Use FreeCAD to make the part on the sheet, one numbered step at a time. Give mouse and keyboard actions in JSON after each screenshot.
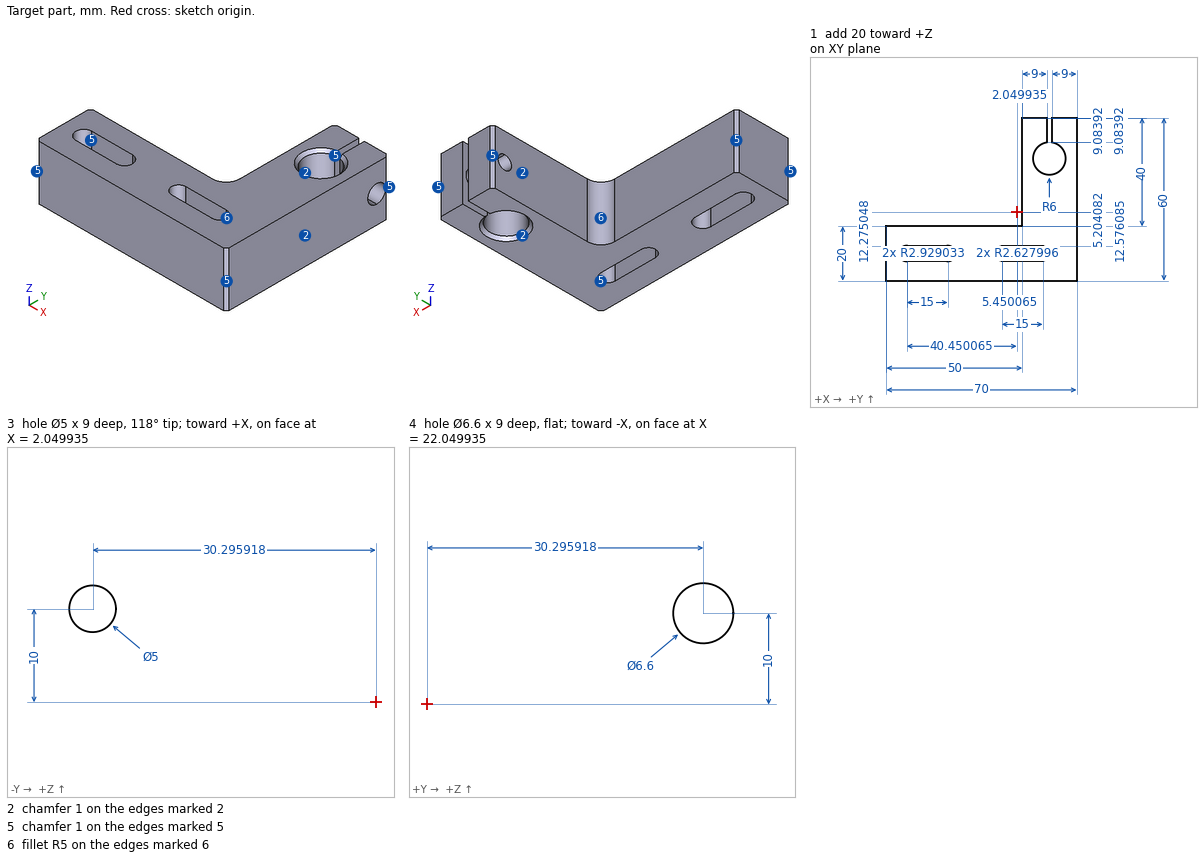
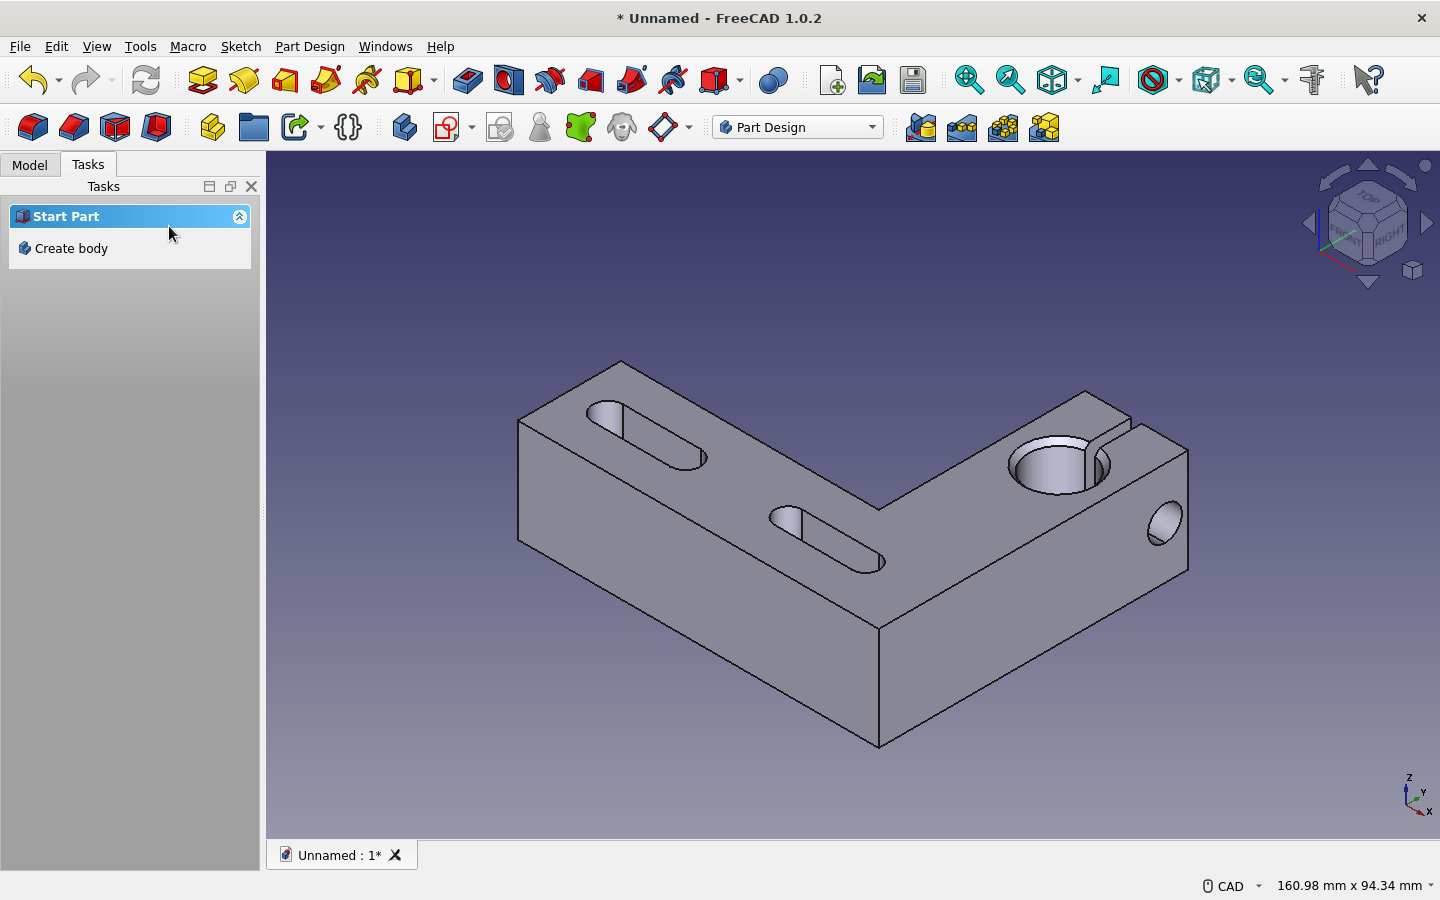
{"action": "left_click", "coordinate": [879, 688]}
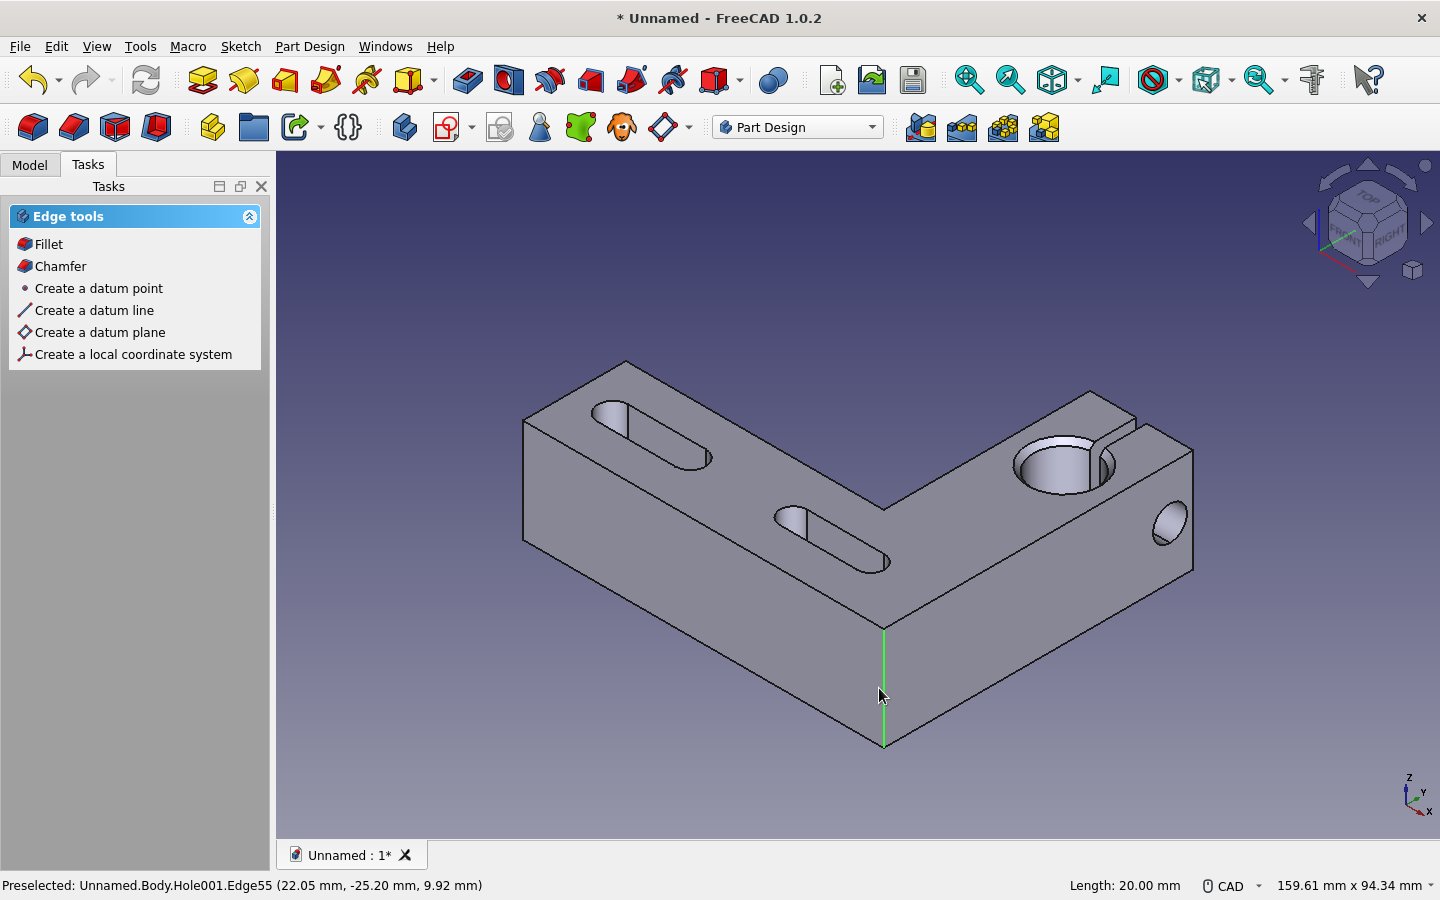
{"action": "key", "text": "2"}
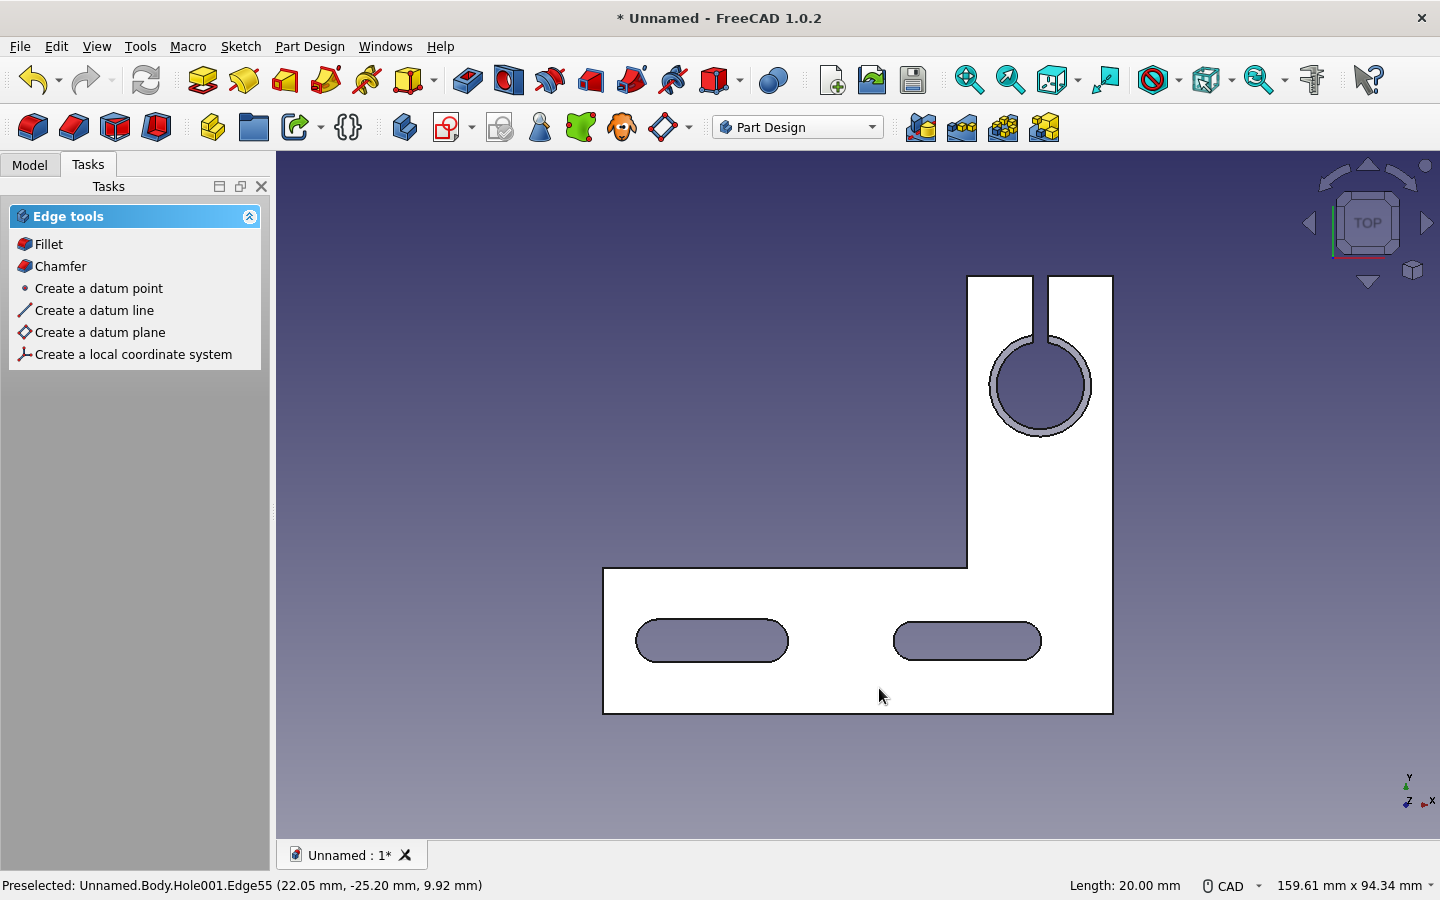
{"action": "key", "text": "0"}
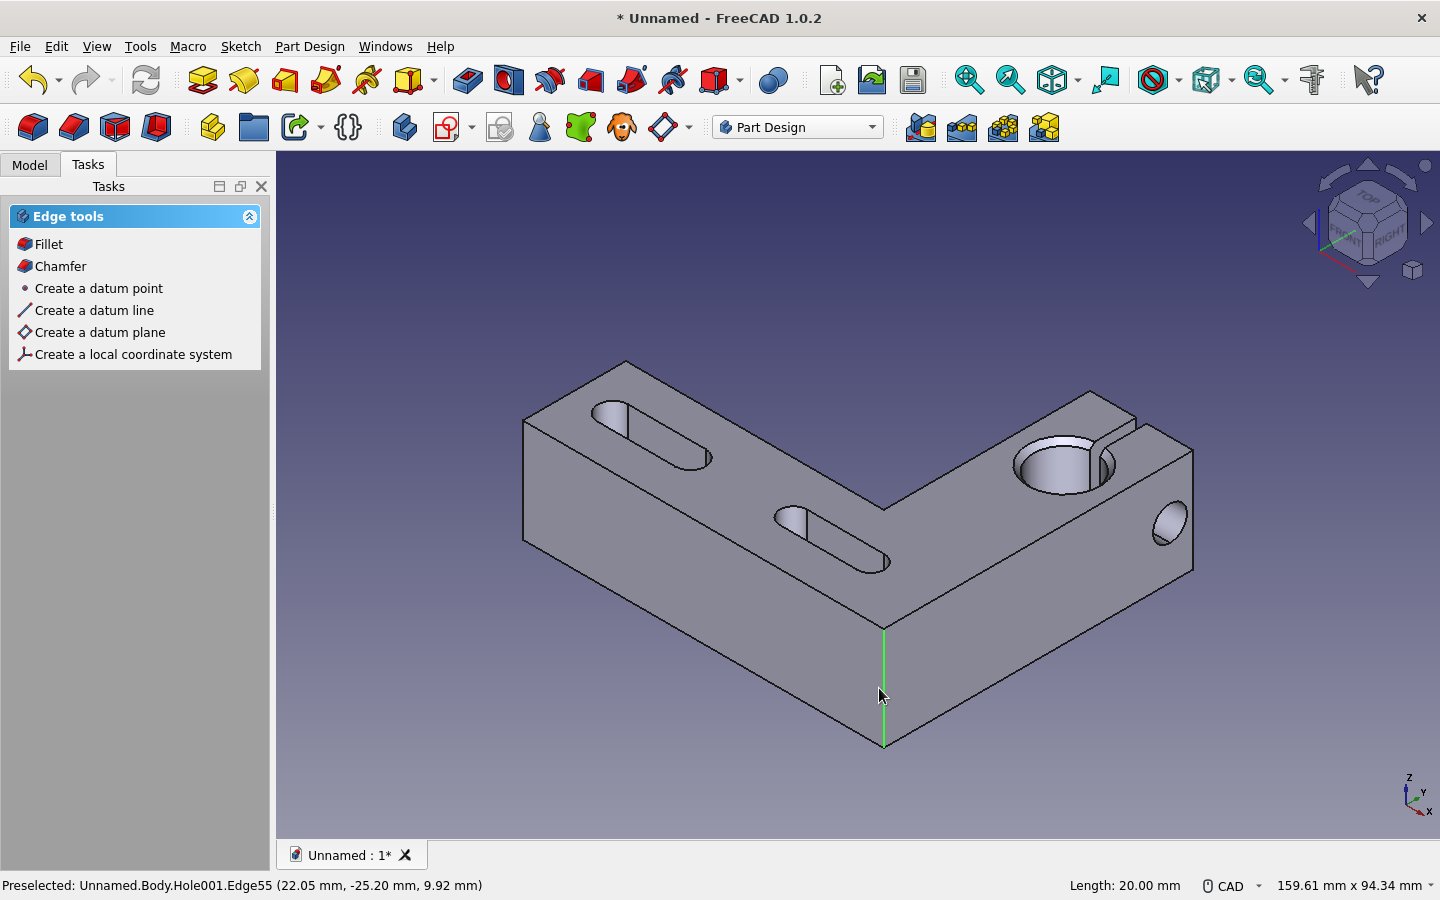
{"action": "key", "text": "1"}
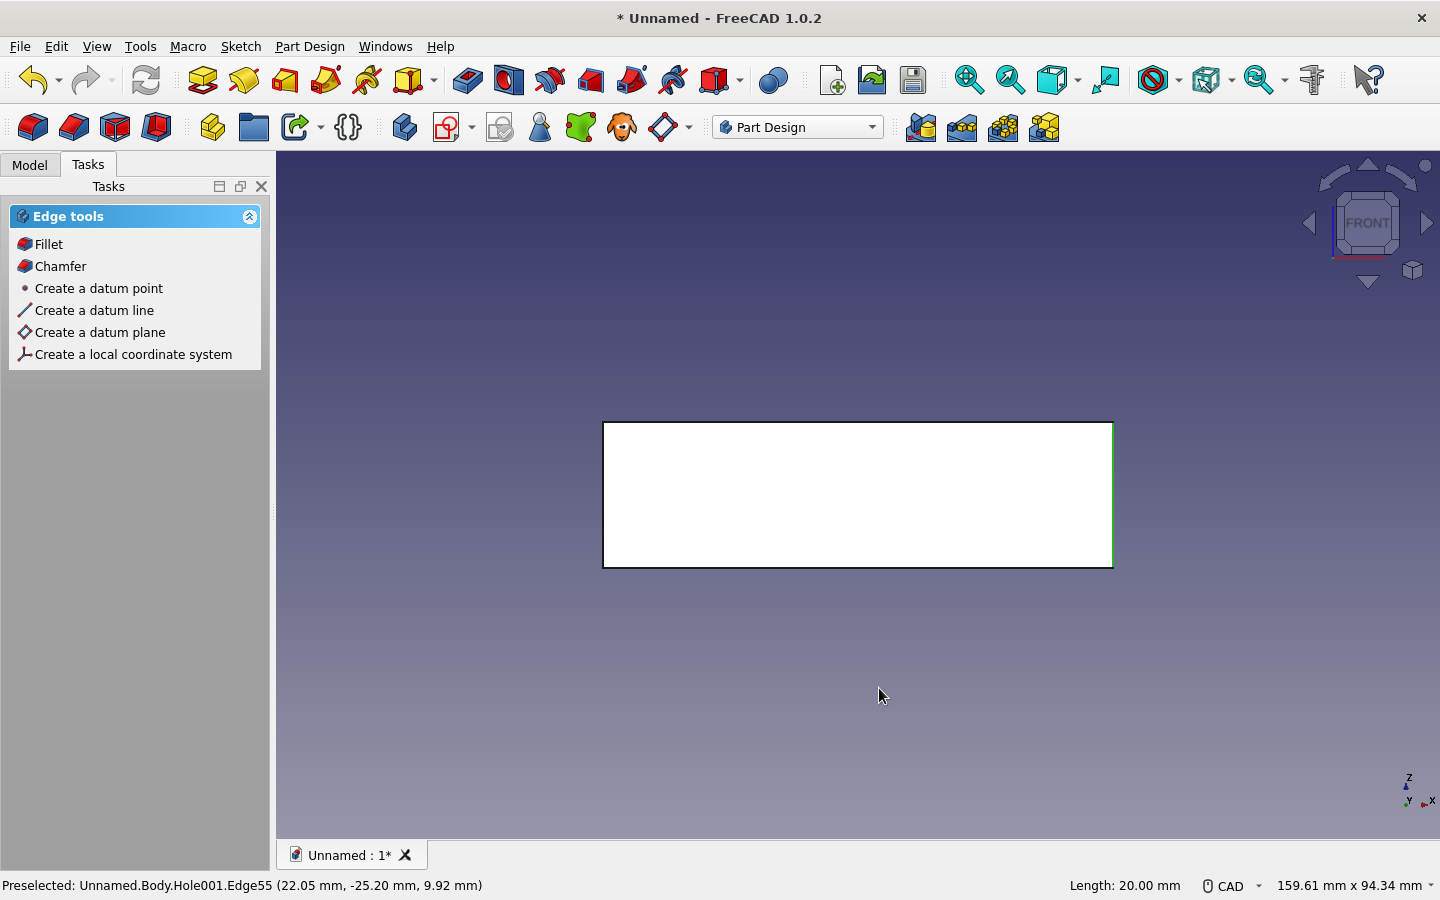
{"action": "left_click", "coordinate": [970, 80]}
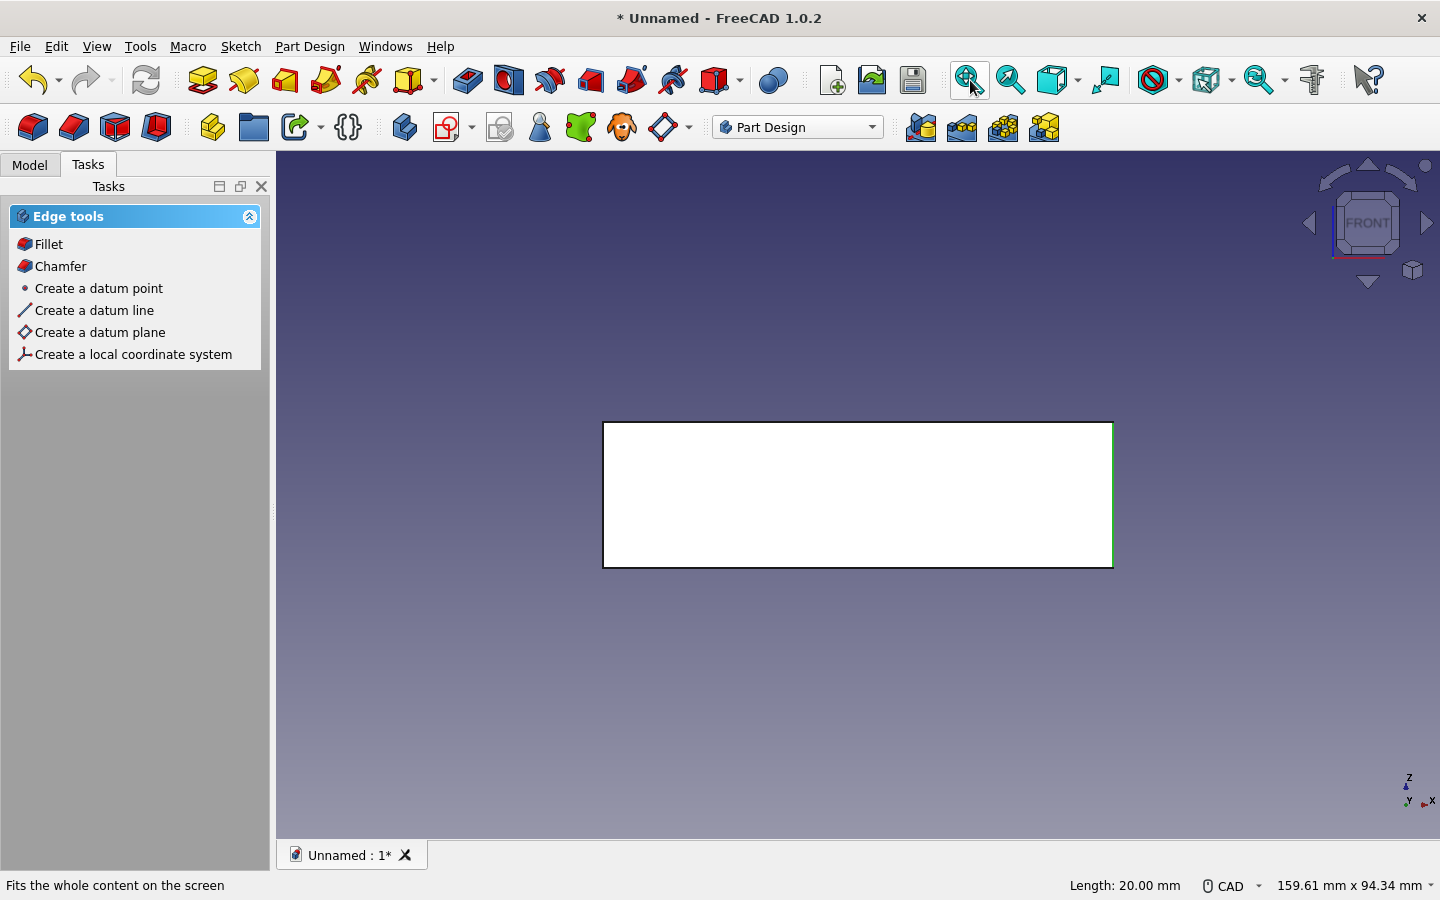
{"action": "left_click", "coordinate": [603, 494], "text": "ctrl"}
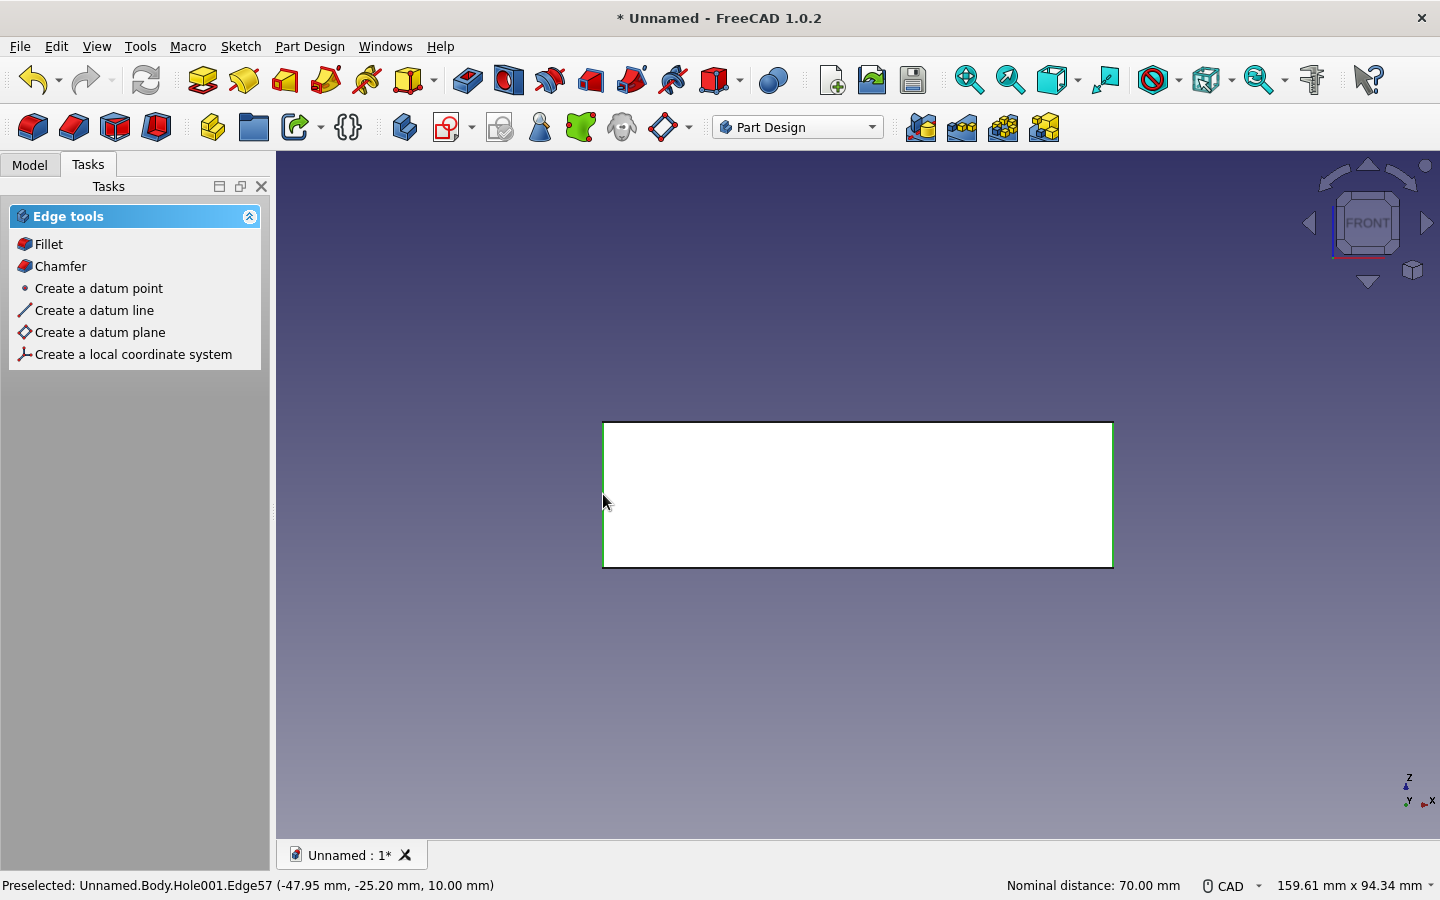
{"action": "key", "text": "3"}